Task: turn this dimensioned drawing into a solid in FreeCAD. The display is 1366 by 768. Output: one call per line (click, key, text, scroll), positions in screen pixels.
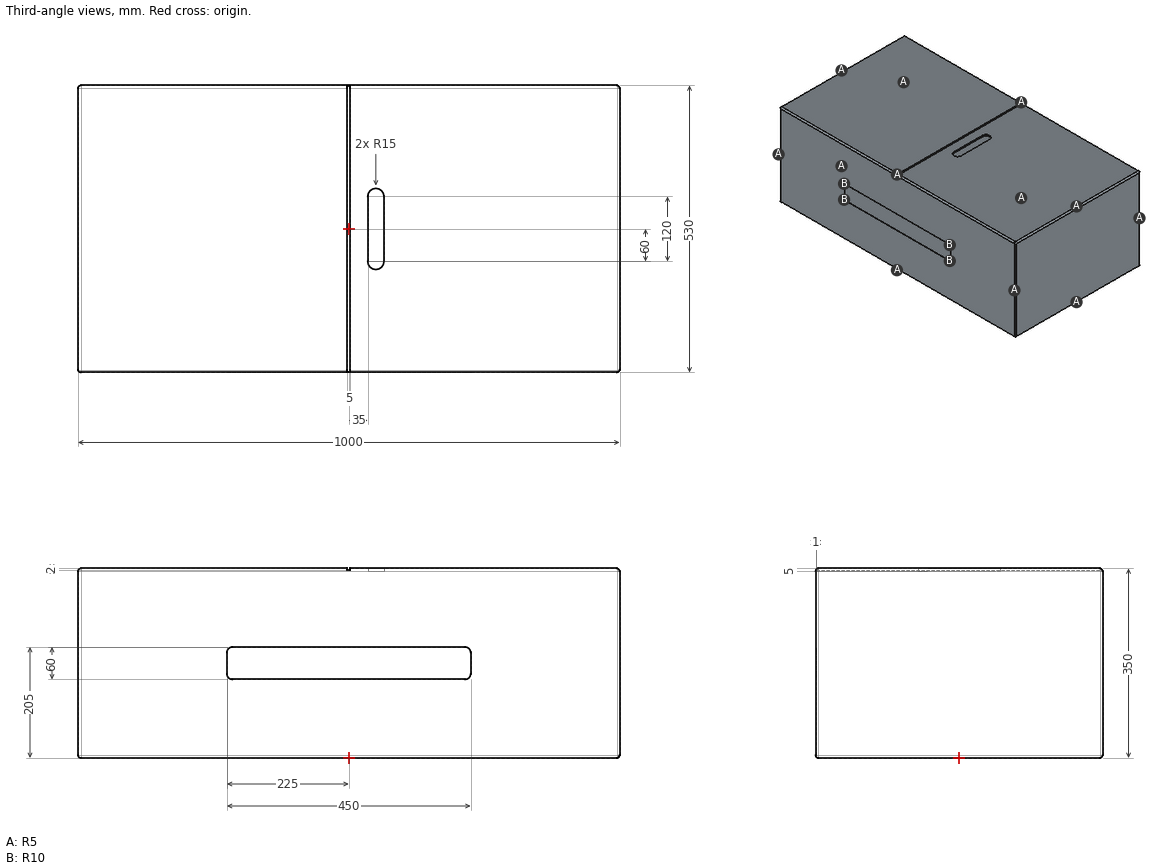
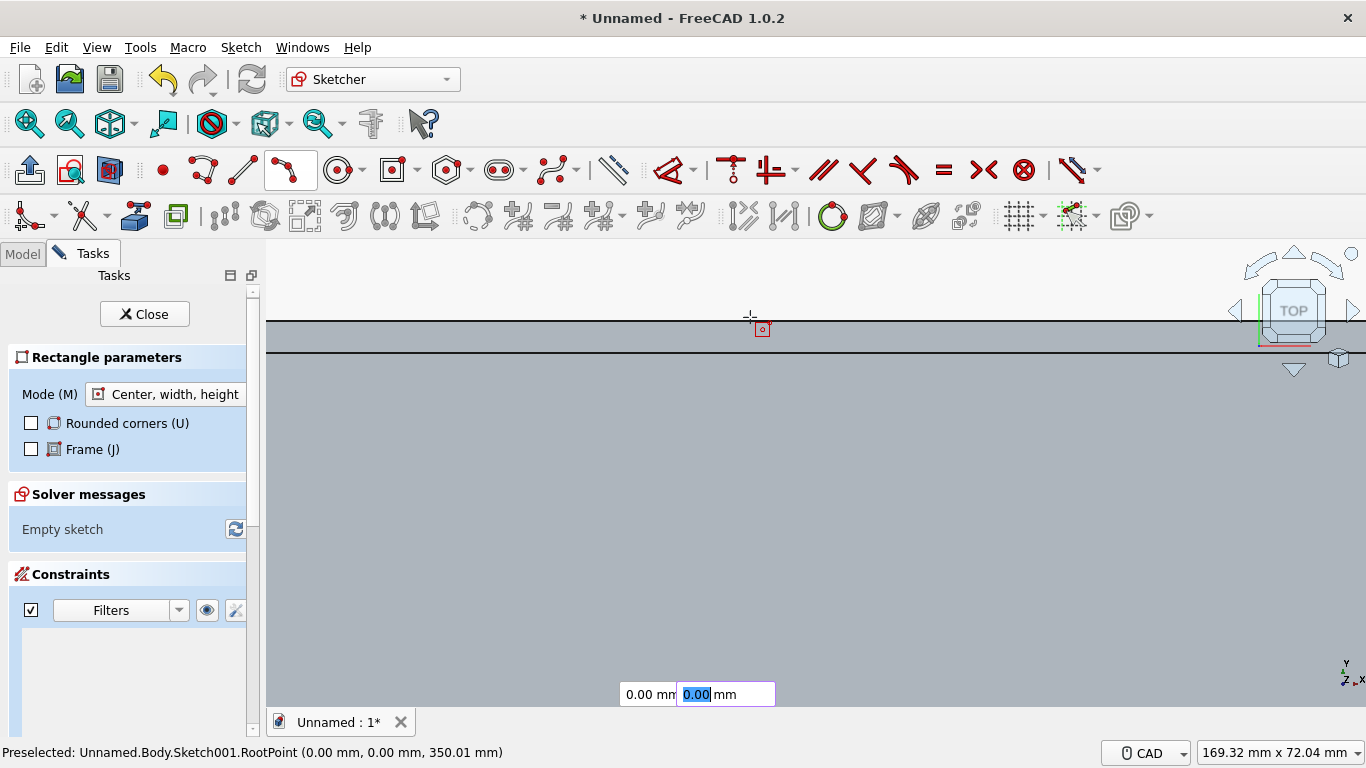
click(742, 321)
key(Escape)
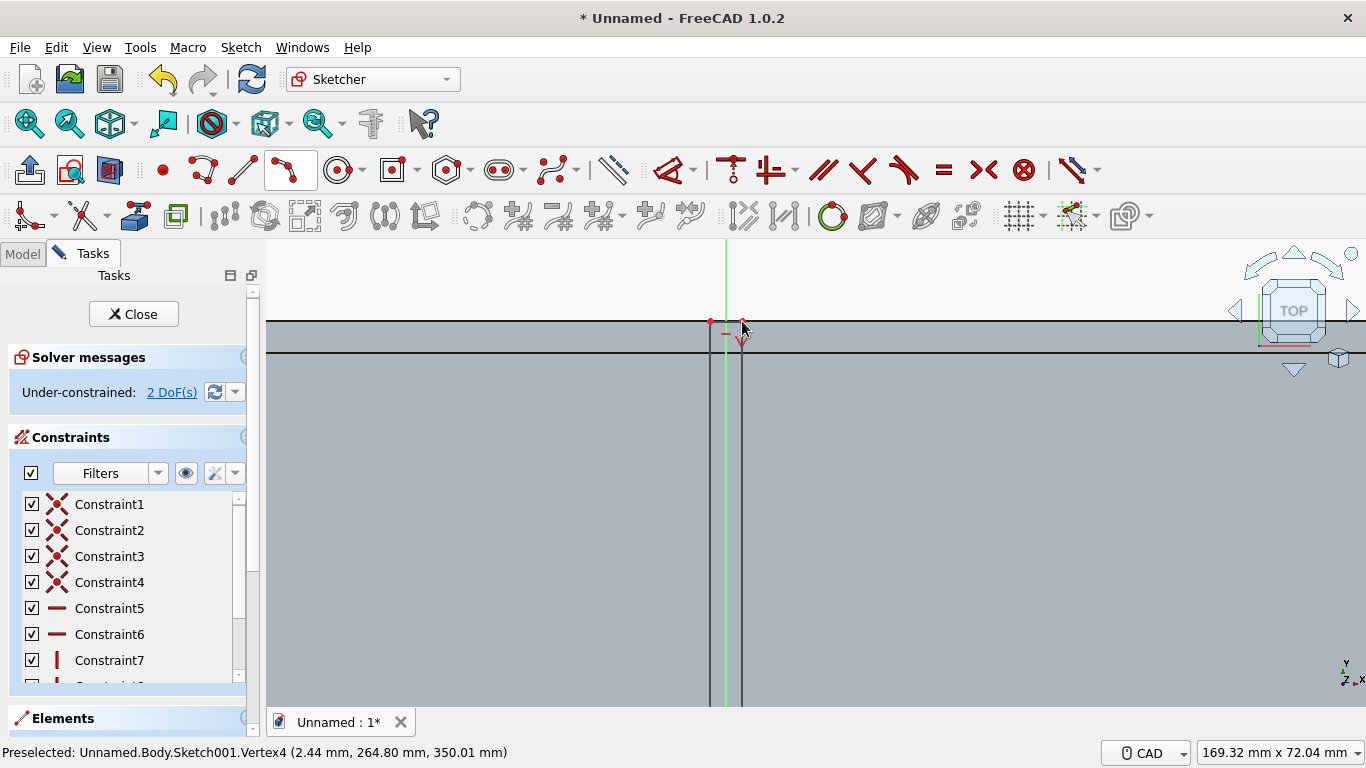
click(668, 170)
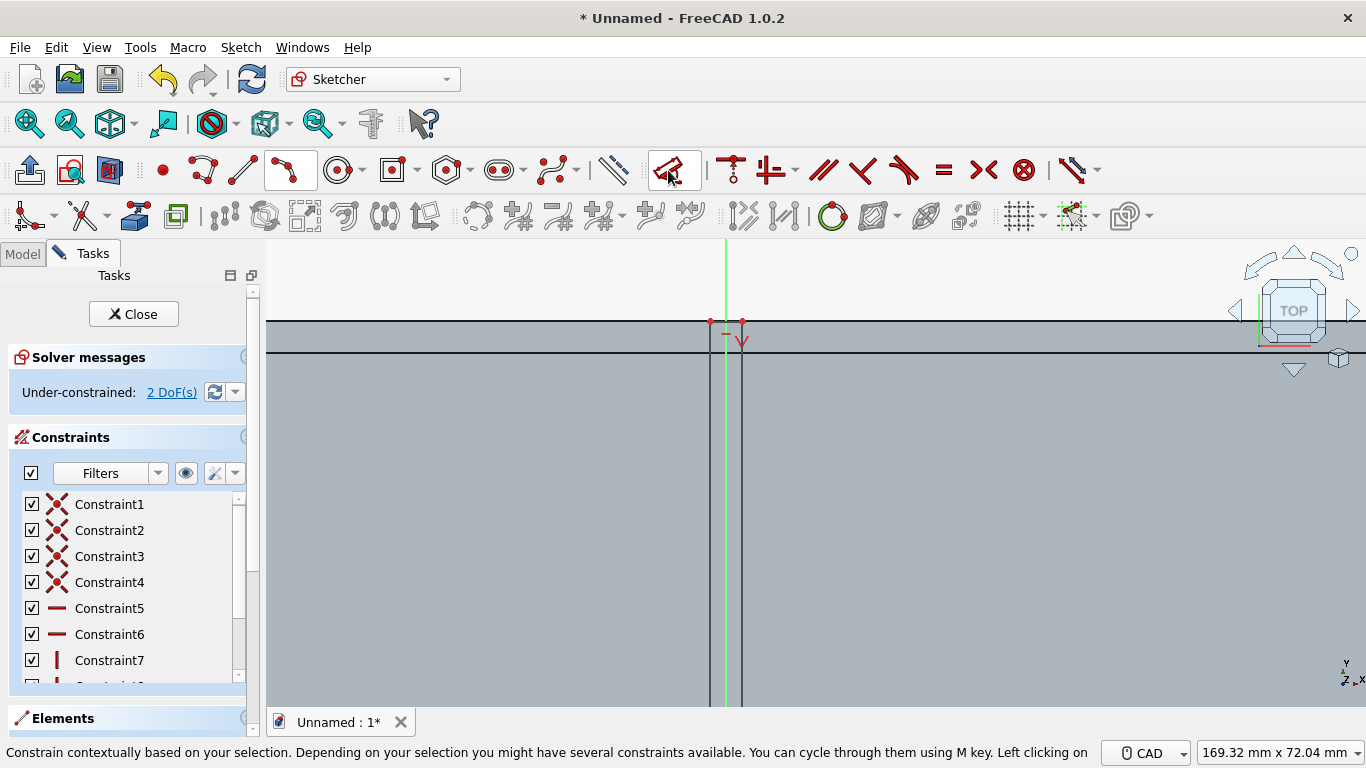
scroll(750, 316, down, 12)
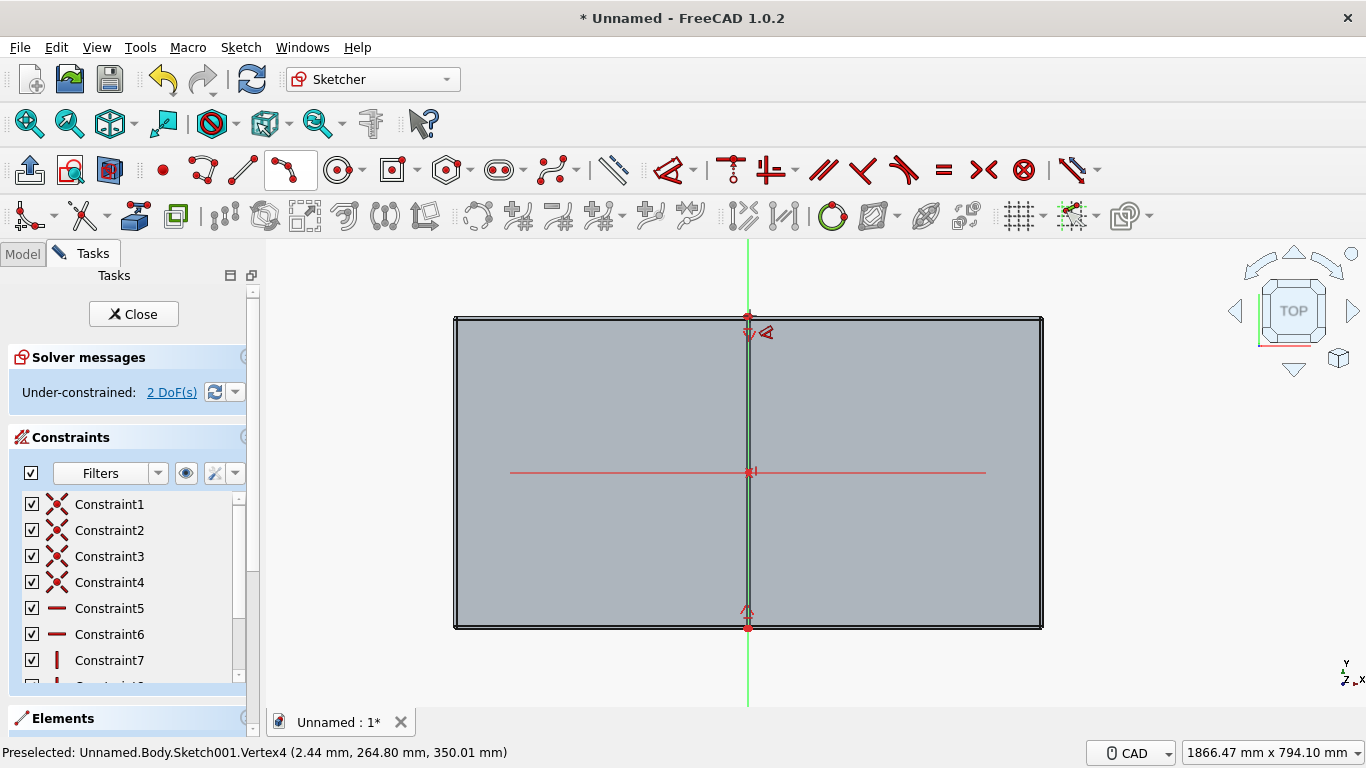
scroll(748, 629, up, 14)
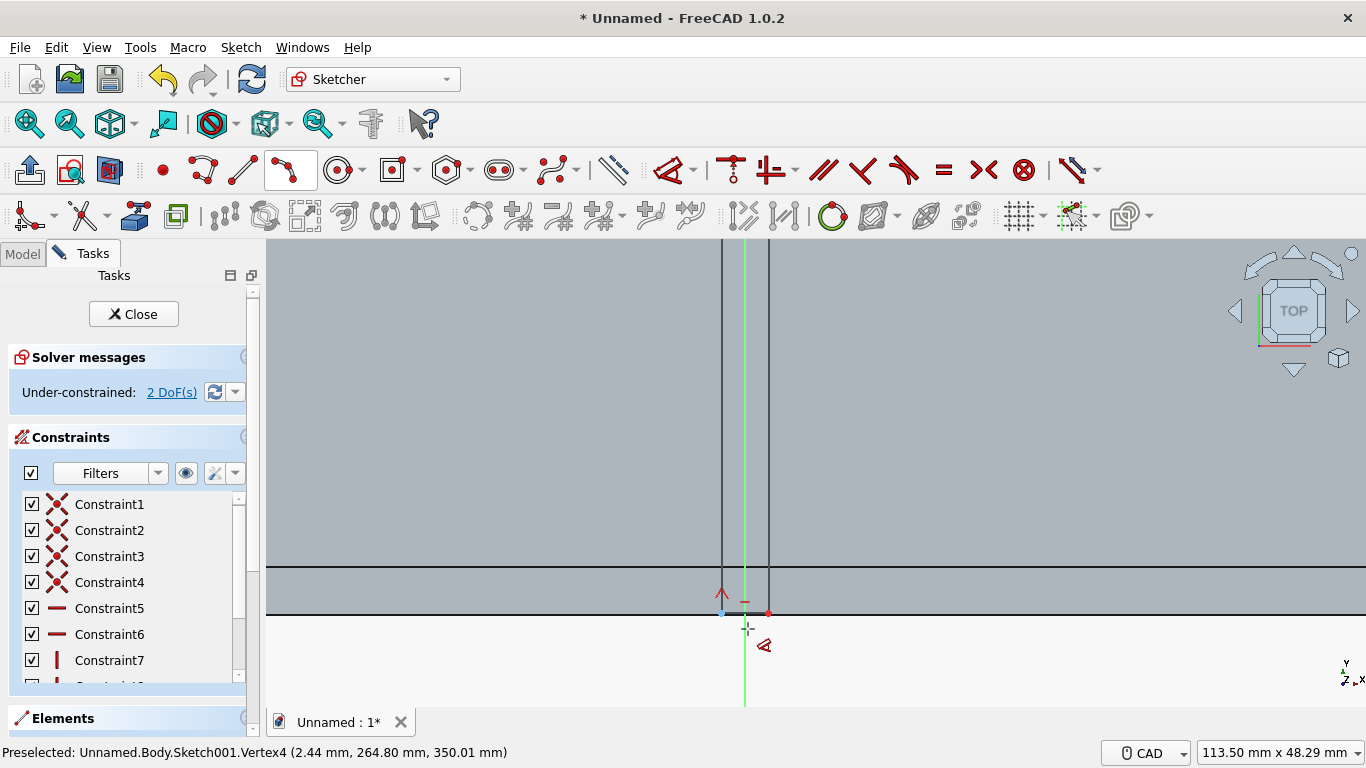
click(740, 613)
click(729, 647)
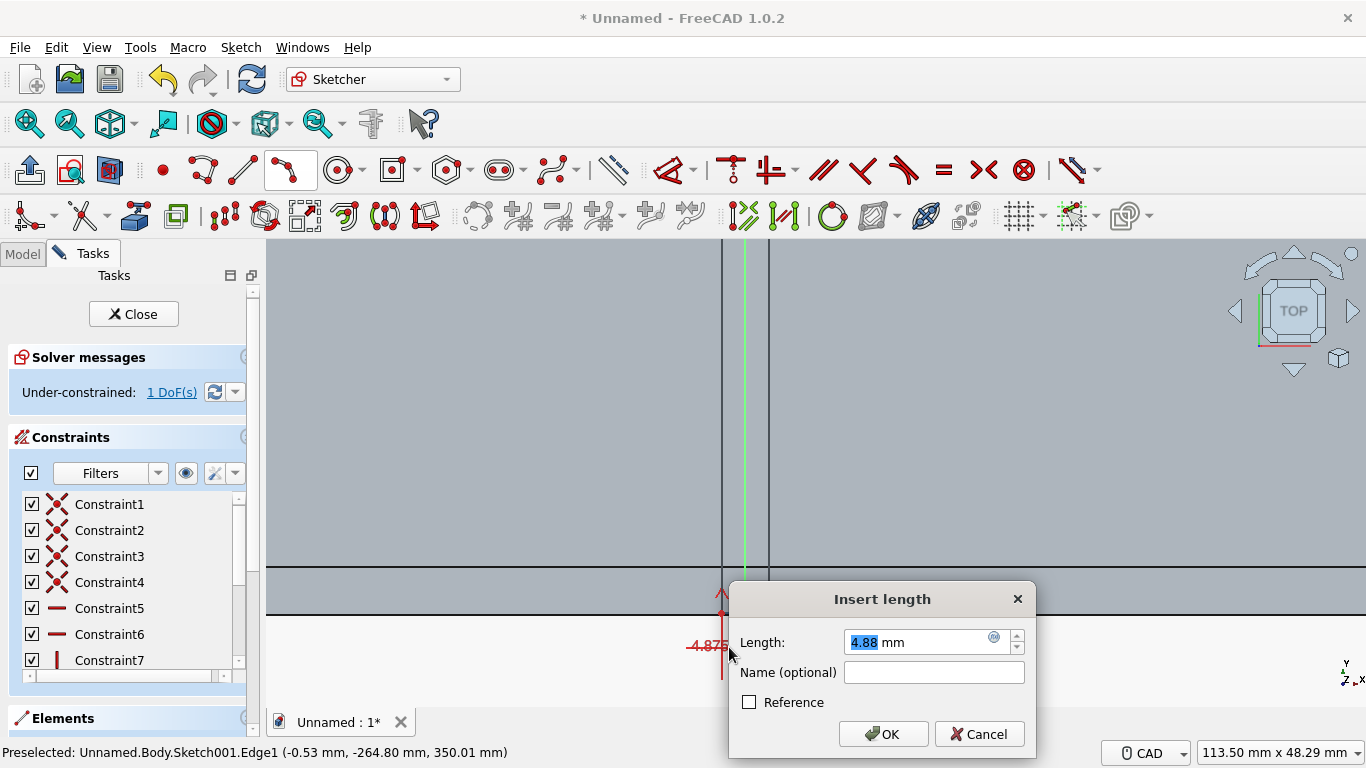
text(5)
key(Return)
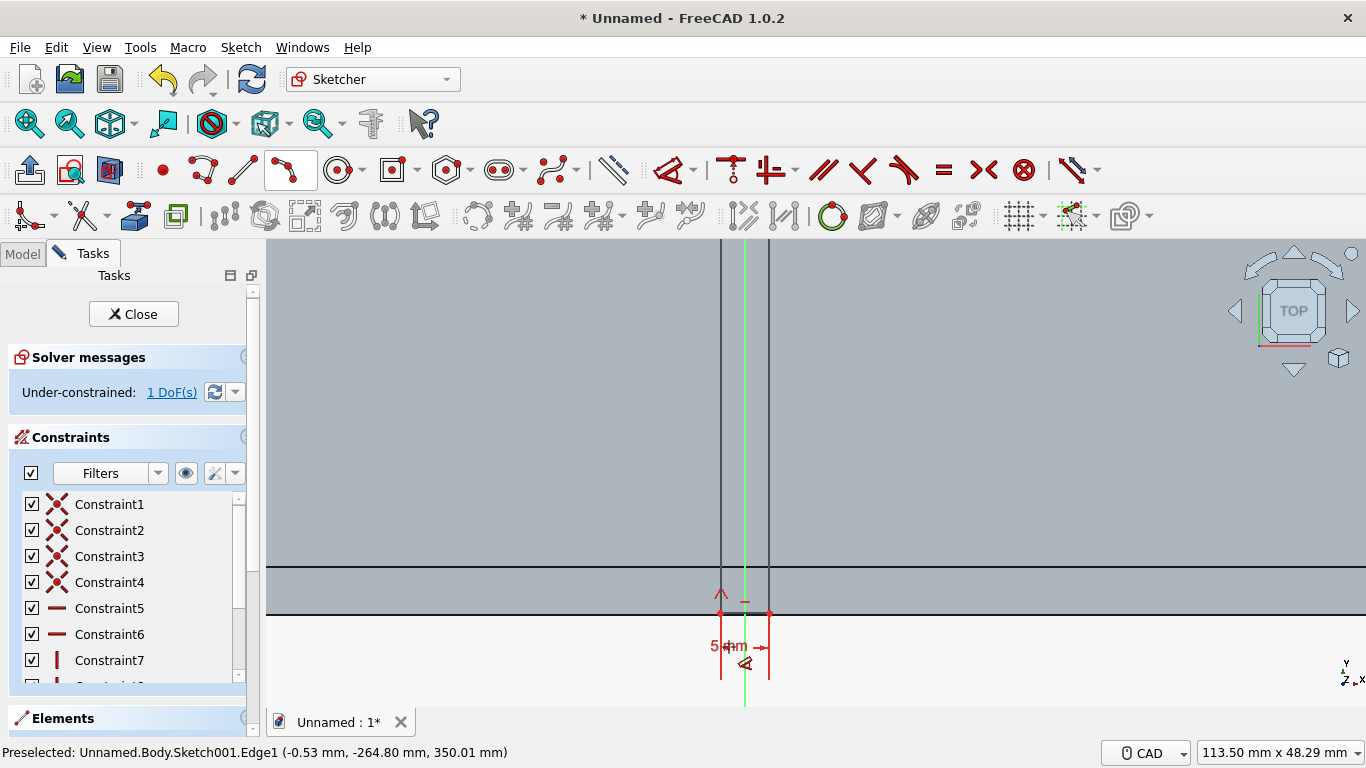
scroll(748, 630, down, 14)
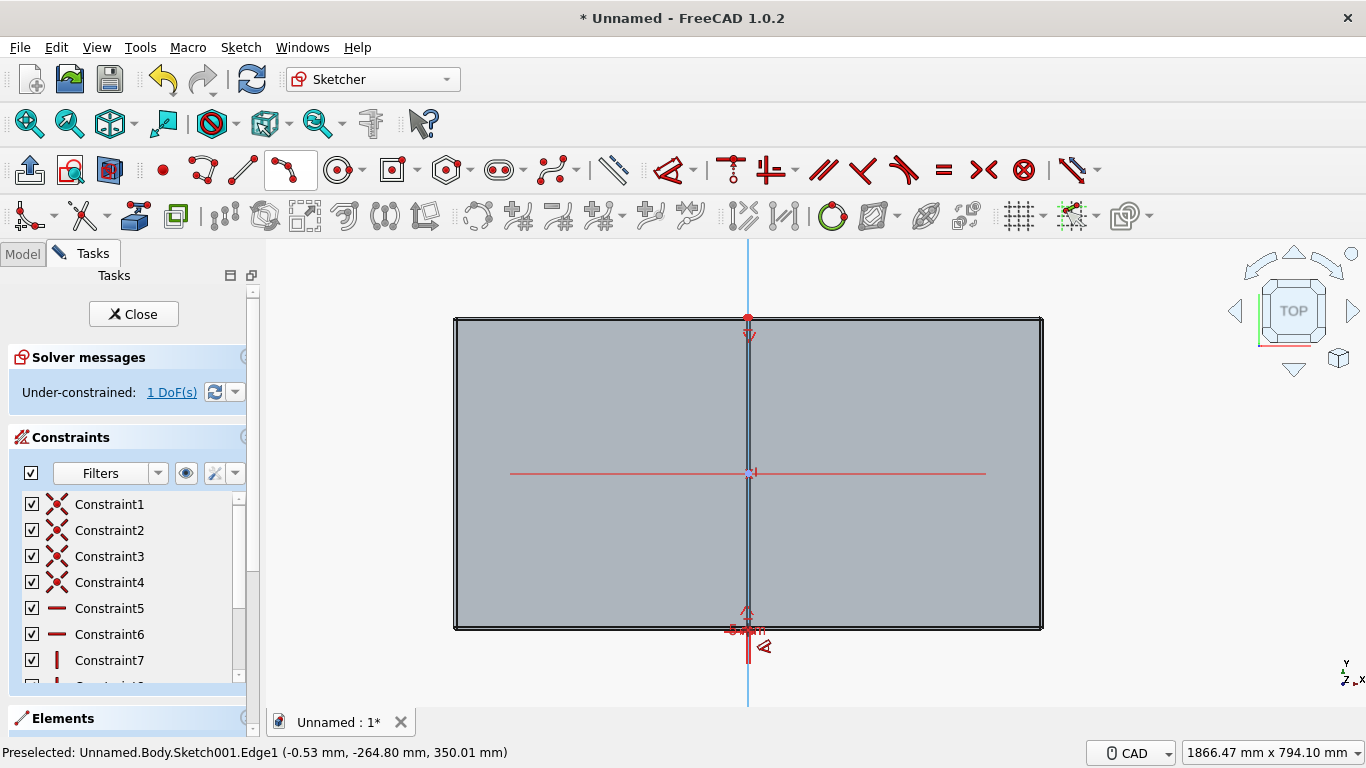
scroll(750, 536, up, 12)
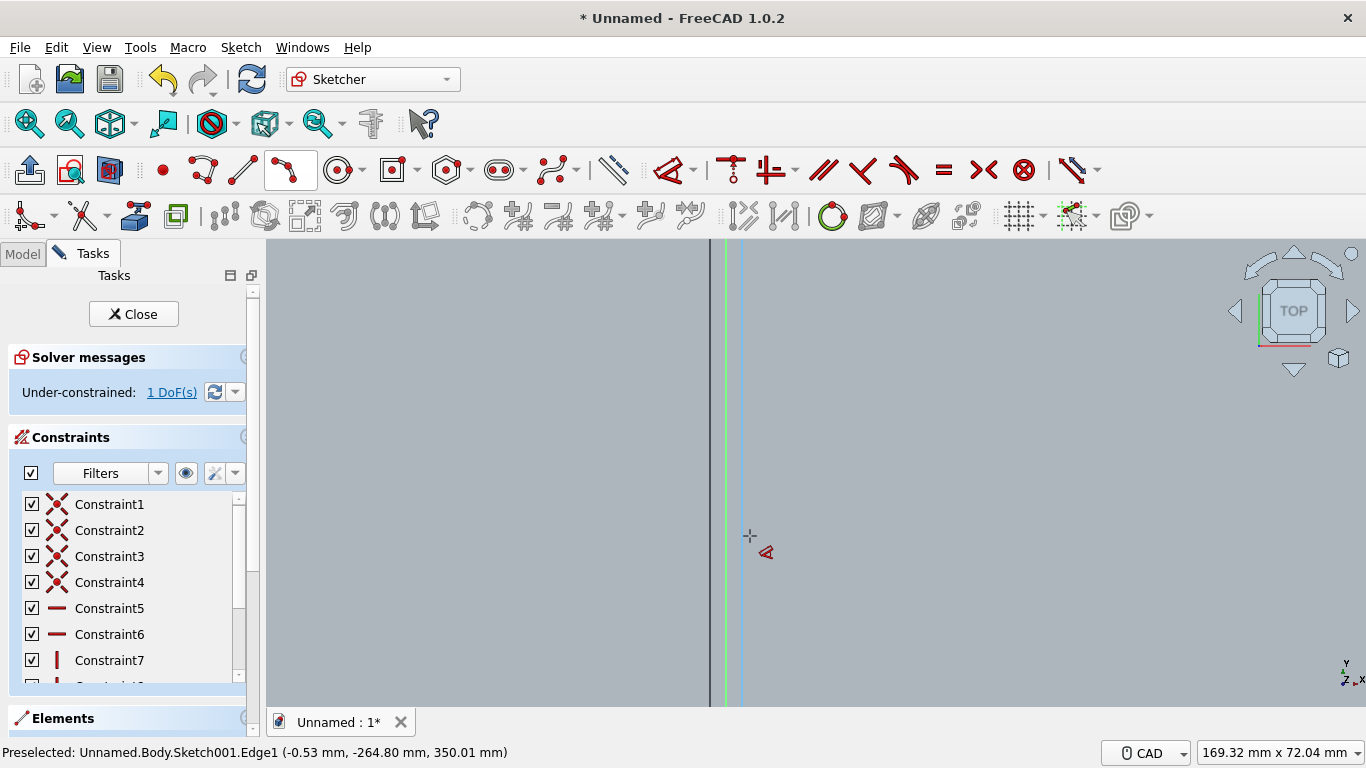
click(742, 531)
click(776, 473)